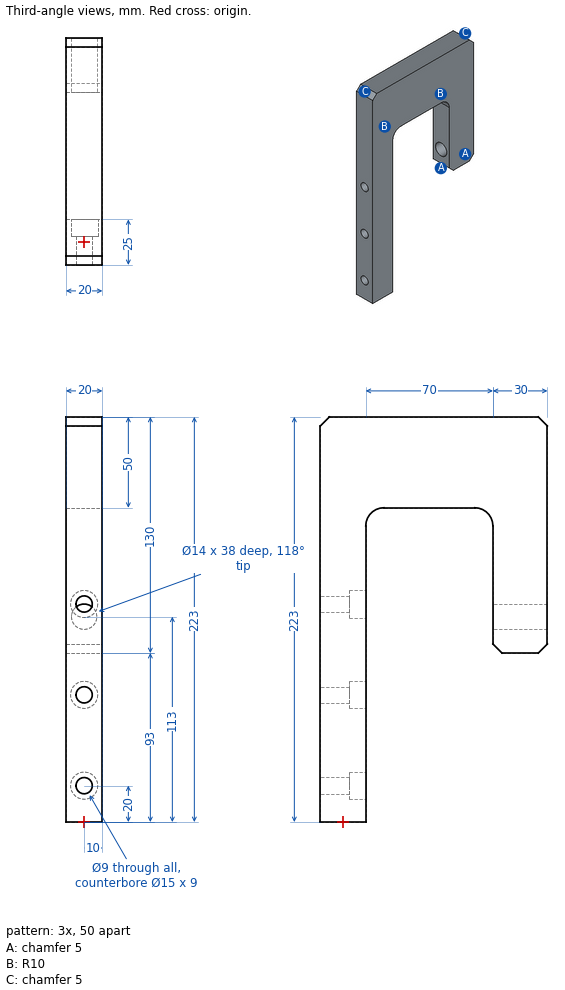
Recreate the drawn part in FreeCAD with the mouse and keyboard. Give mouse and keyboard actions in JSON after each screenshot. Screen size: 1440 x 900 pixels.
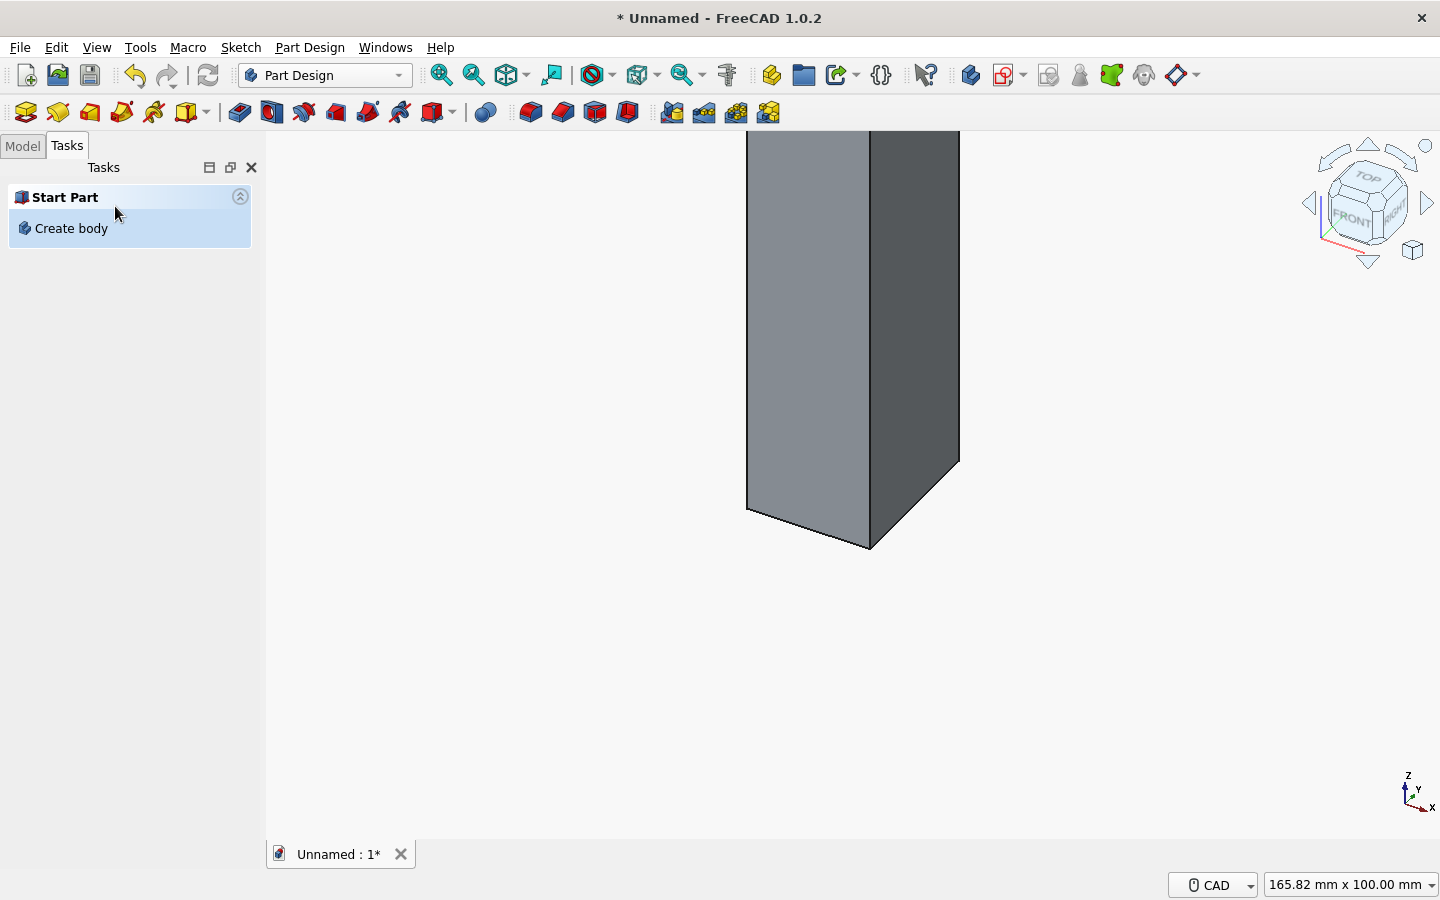
{"action": "left_click", "coordinate": [442, 76]}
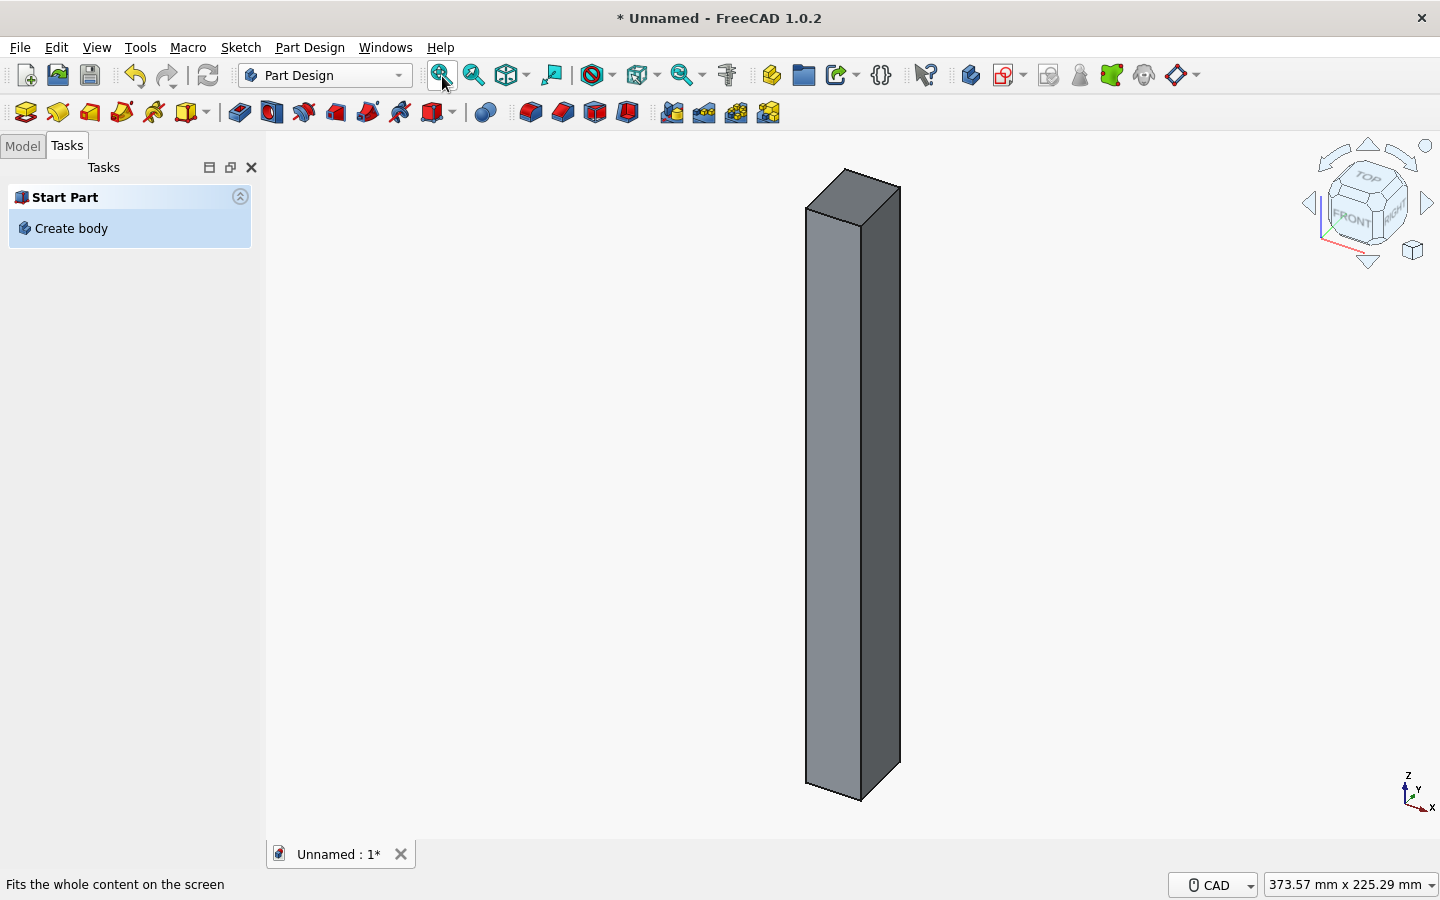
{"action": "key", "text": "4"}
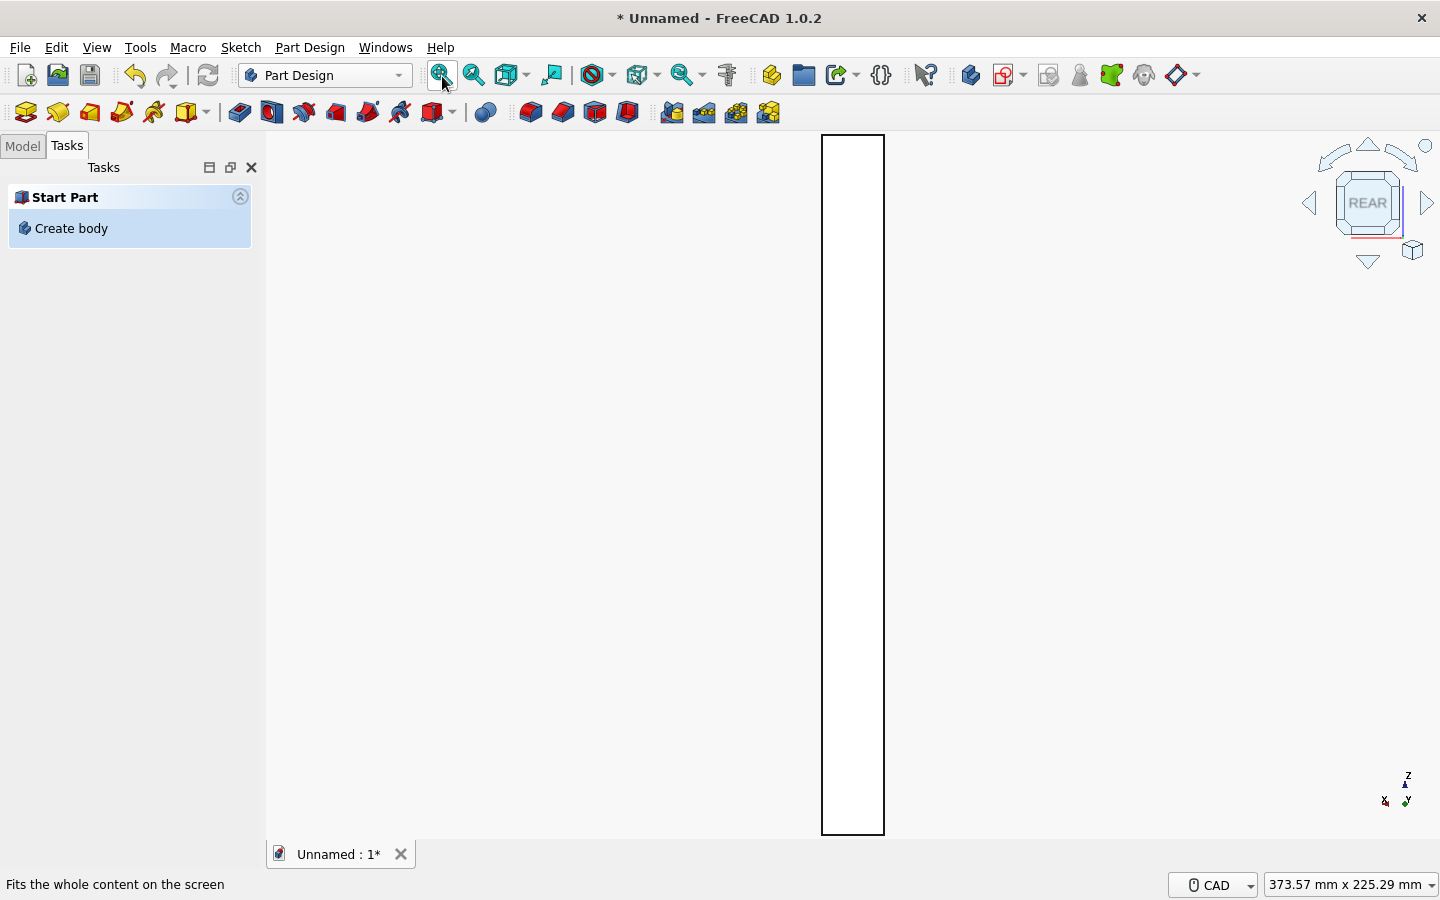
{"action": "left_click", "coordinate": [853, 184]}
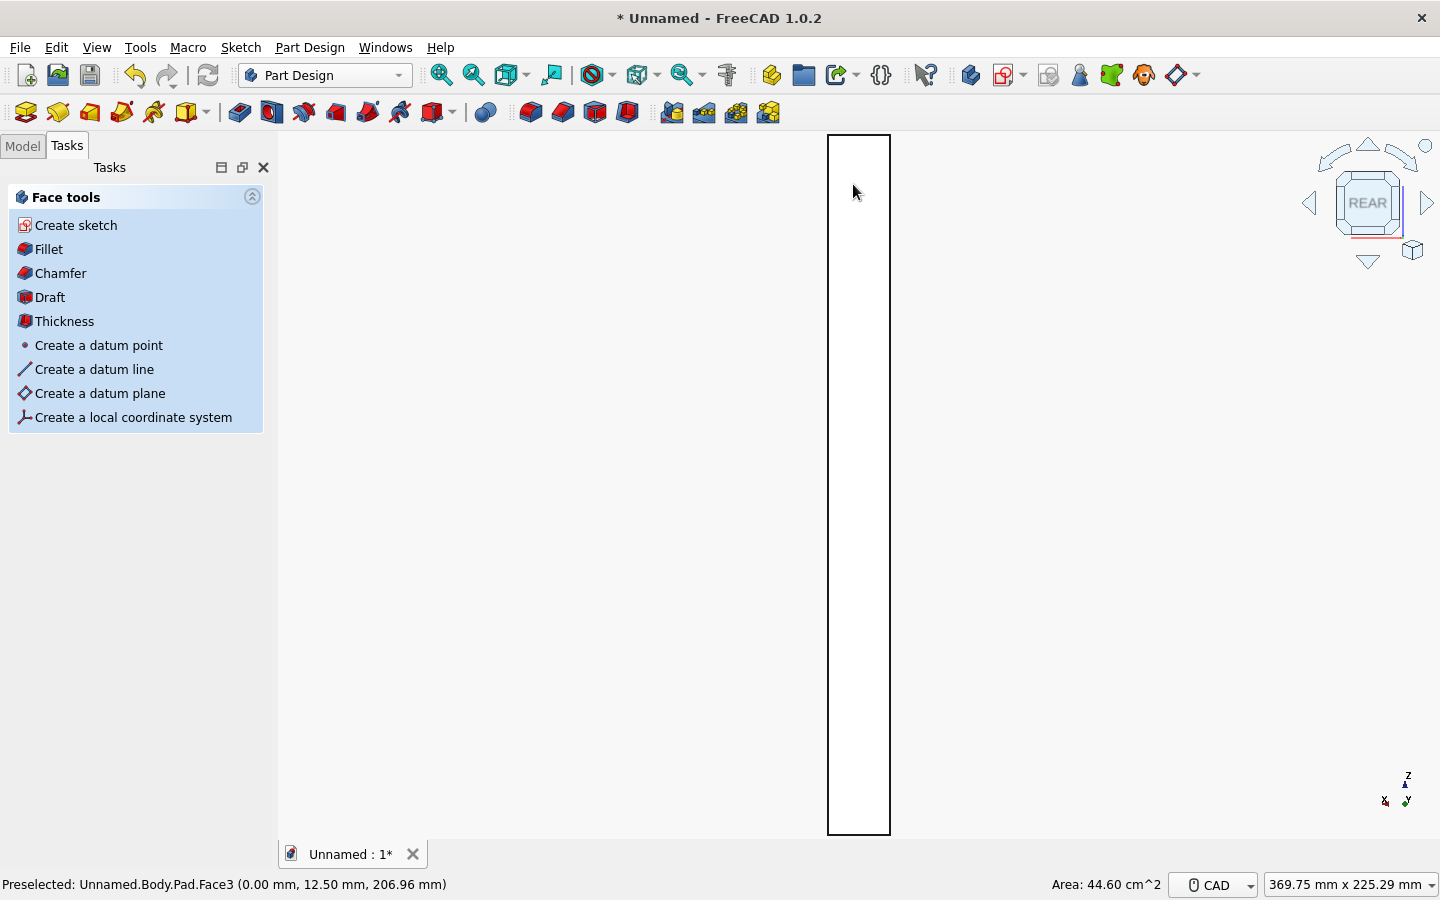
{"action": "left_click", "coordinate": [1004, 76]}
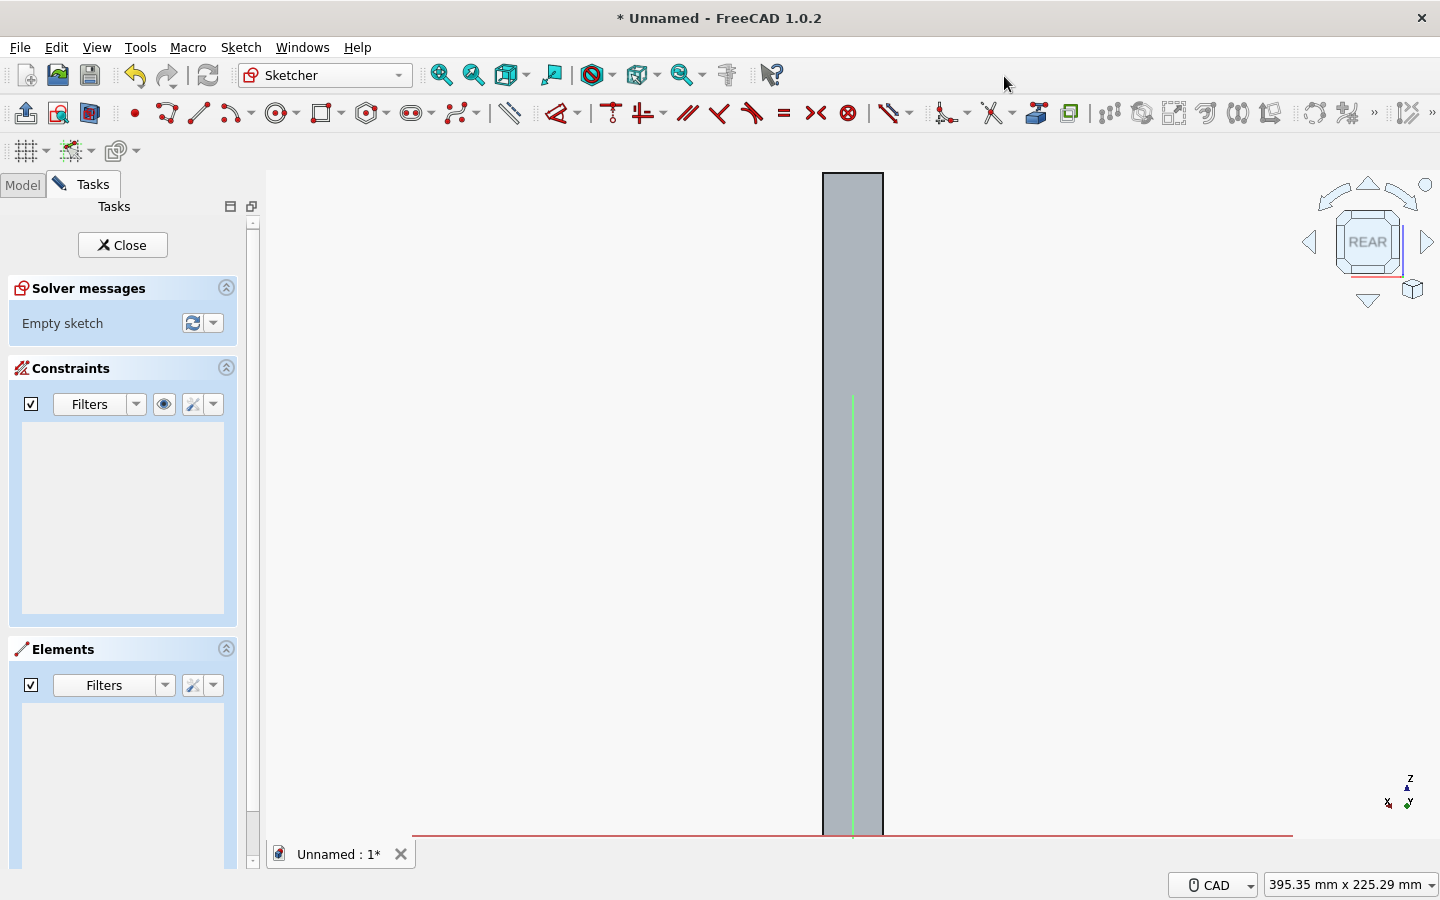
{"action": "scroll", "coordinate": [857, 794], "scroll_direction": "up", "scroll_amount": 14}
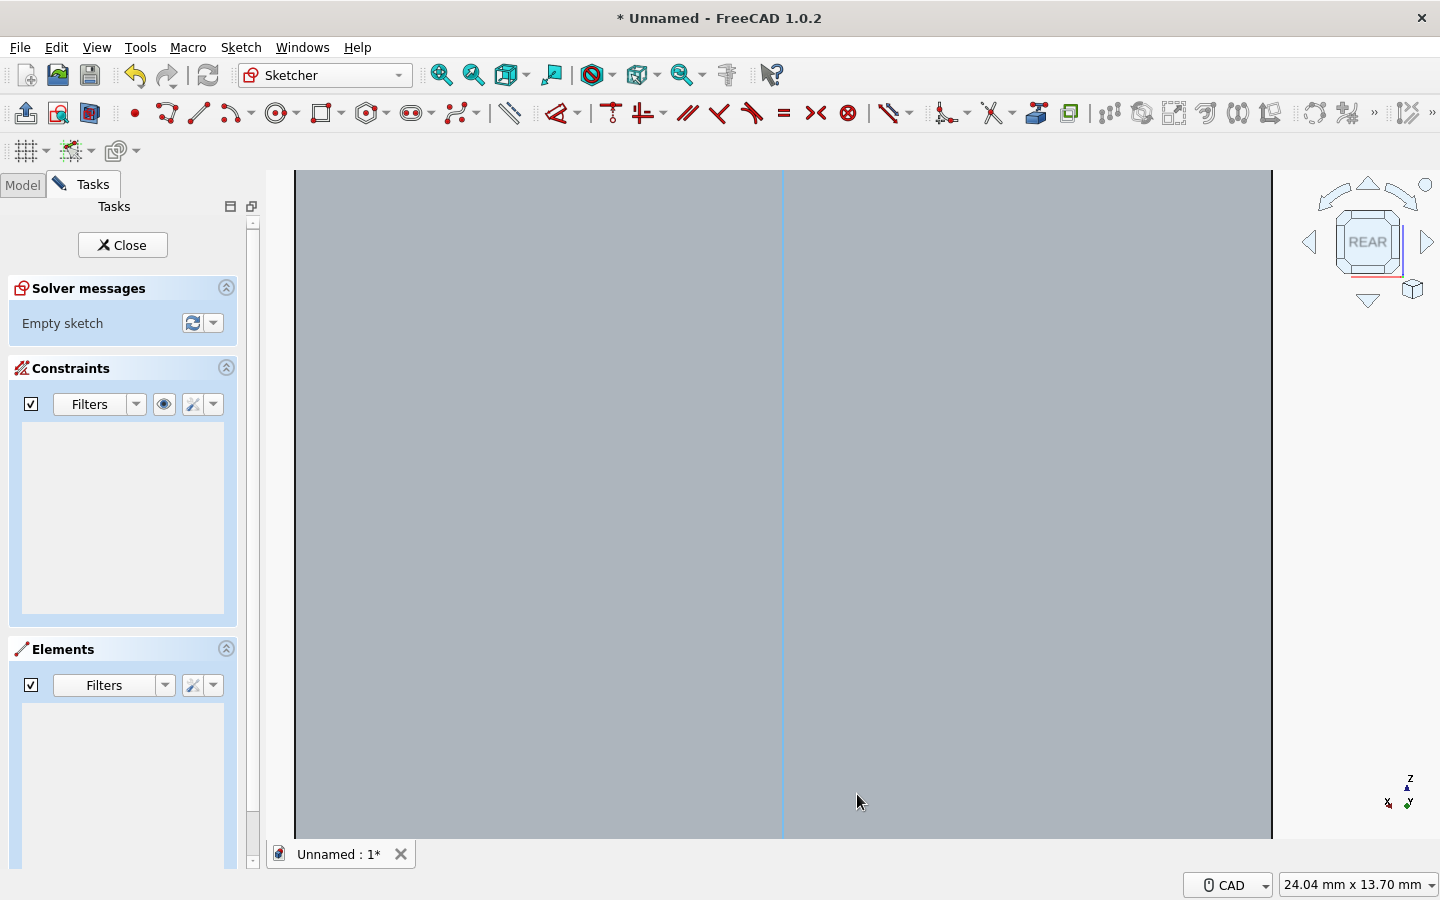
{"action": "left_click", "coordinate": [276, 114]}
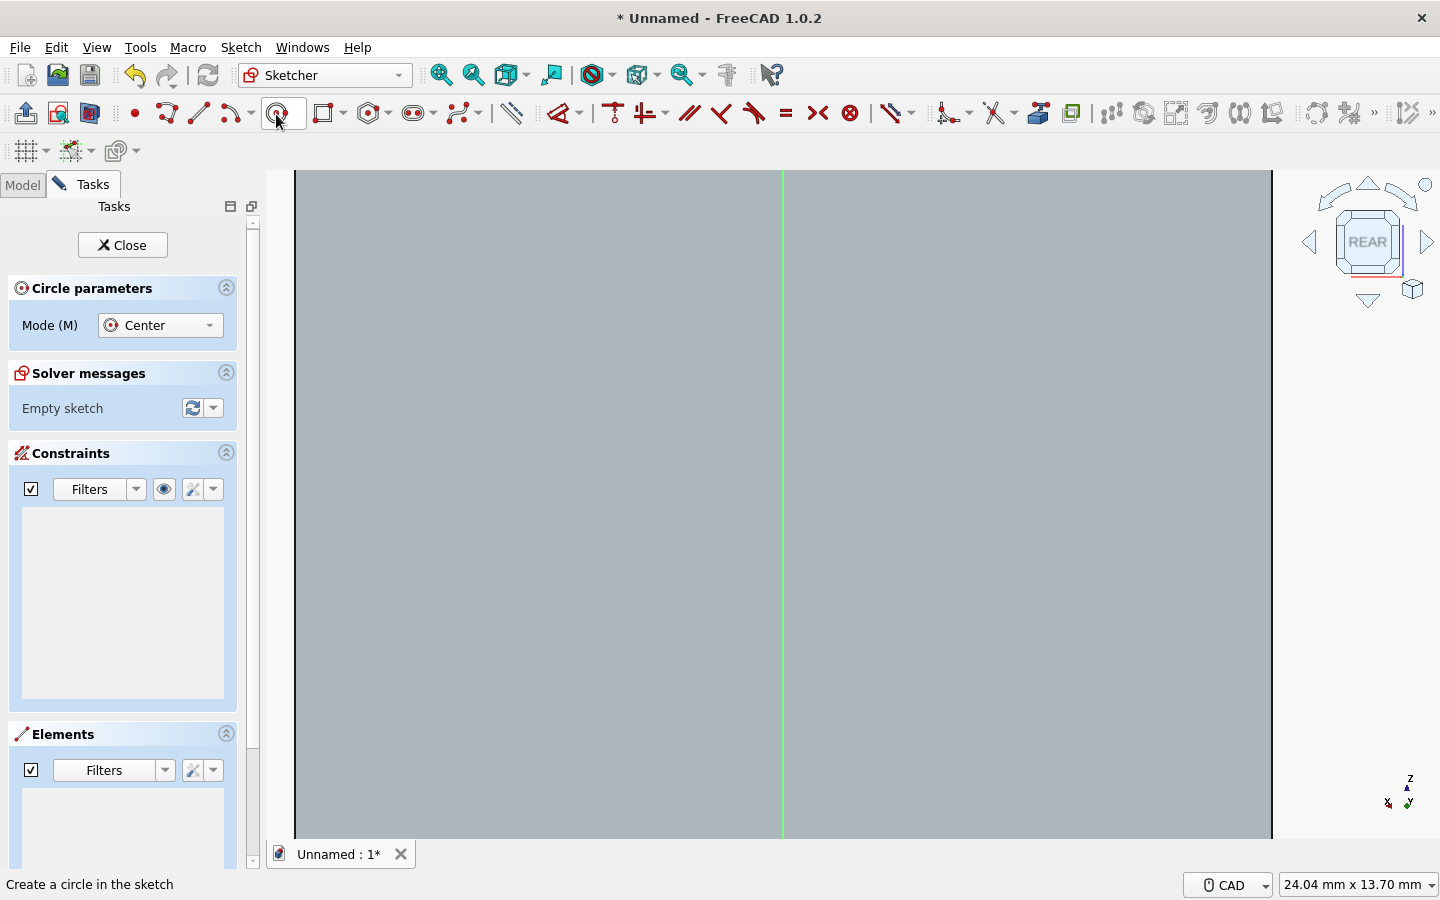
{"action": "left_click", "coordinate": [783, 487]}
{"action": "left_click", "coordinate": [939, 332]}
{"action": "key", "text": "Escape"}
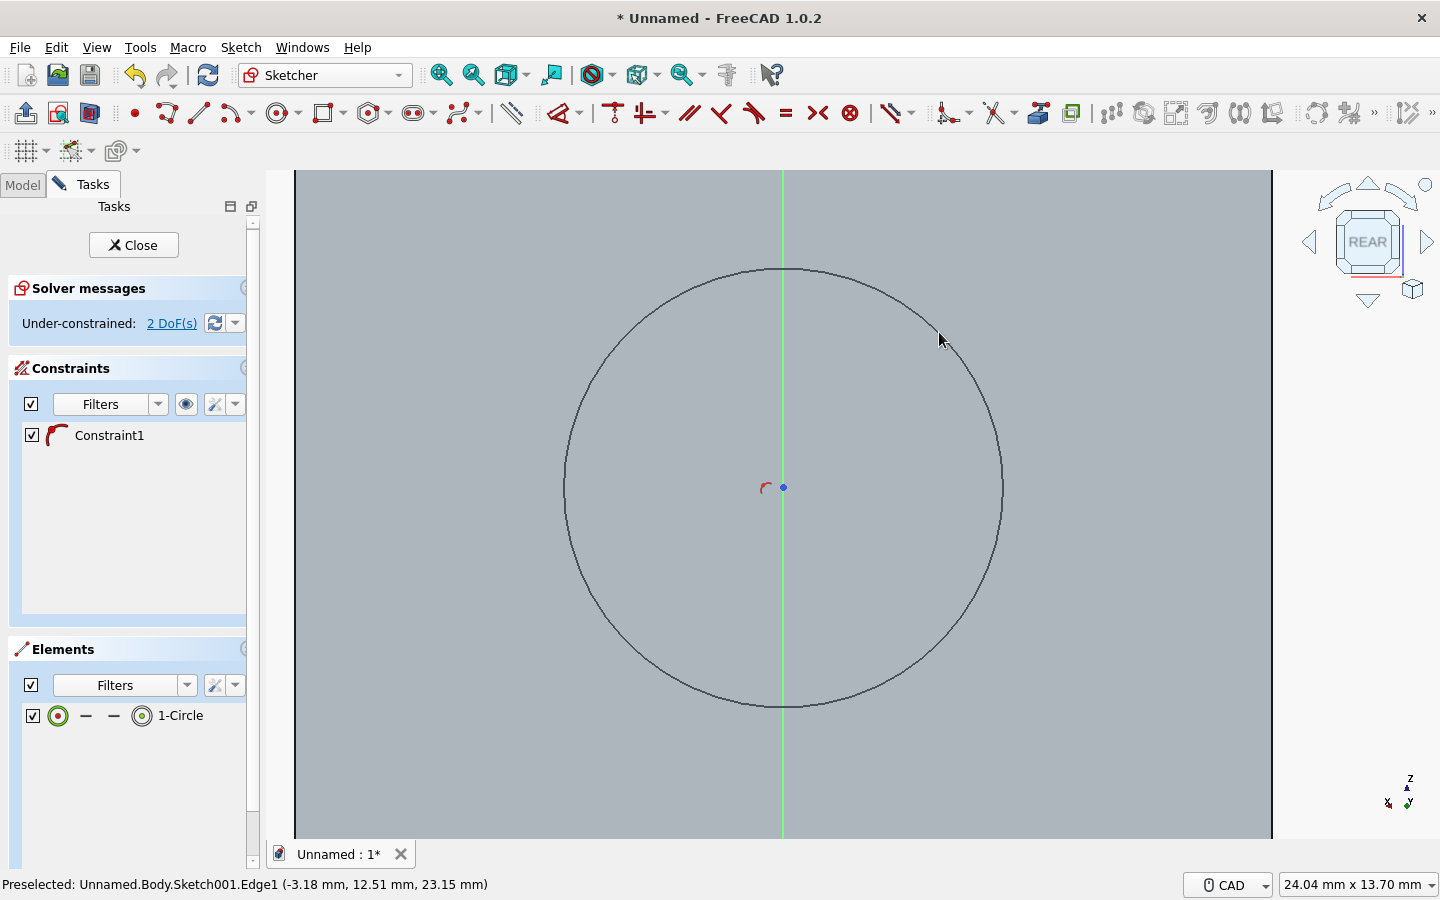
{"action": "left_click", "coordinate": [558, 114]}